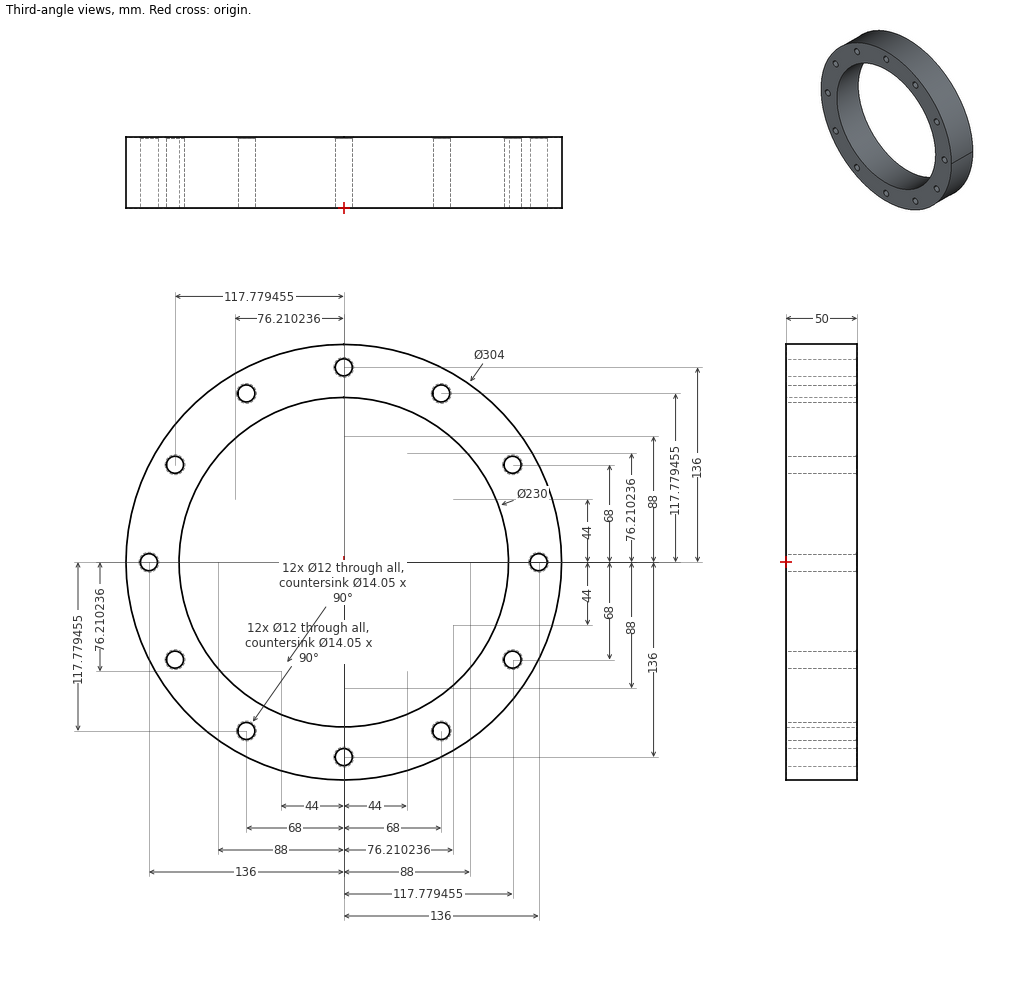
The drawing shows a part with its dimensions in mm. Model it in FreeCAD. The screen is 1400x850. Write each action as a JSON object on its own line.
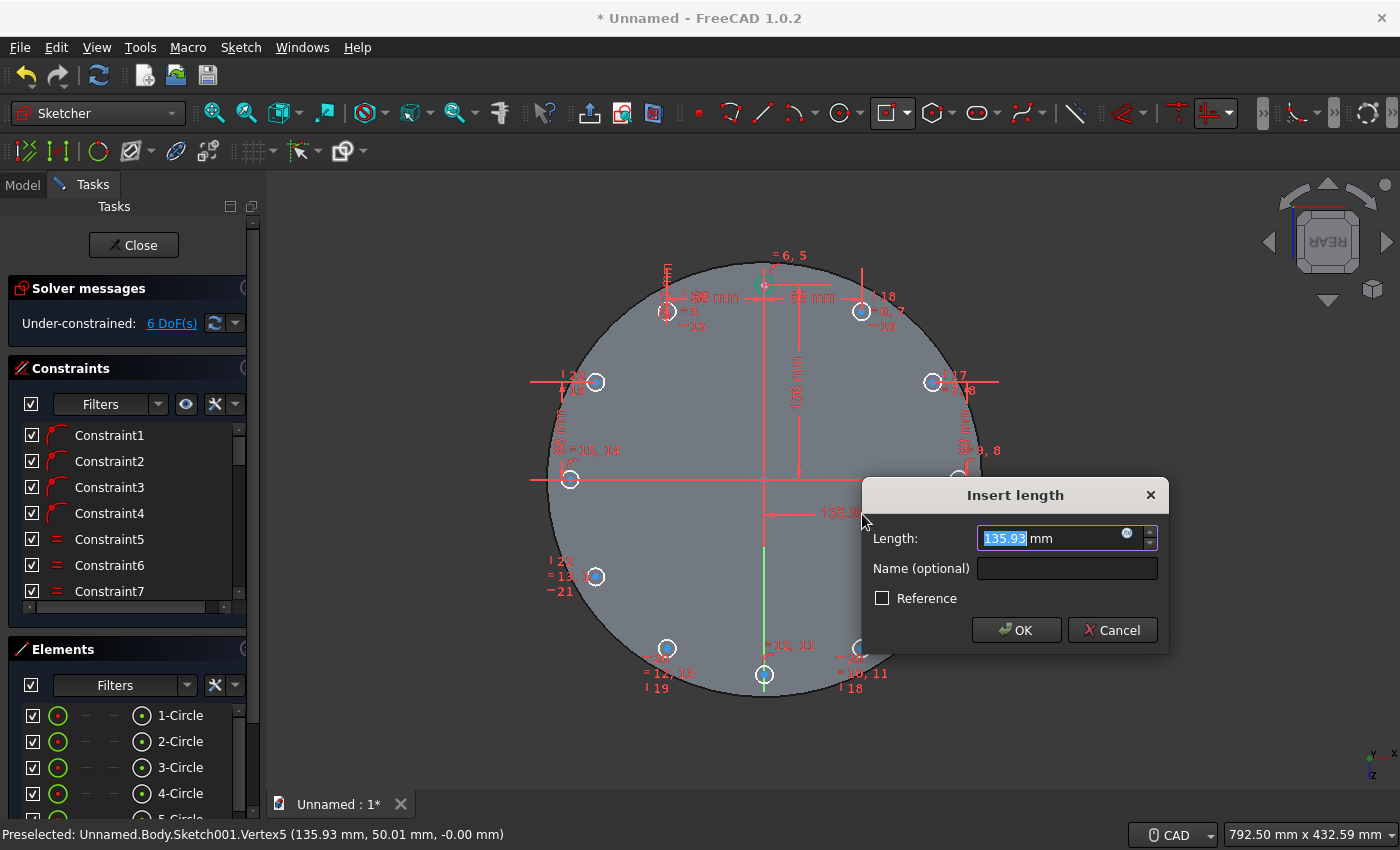
{"action": "type", "text": "136"}
{"action": "key", "text": "Return"}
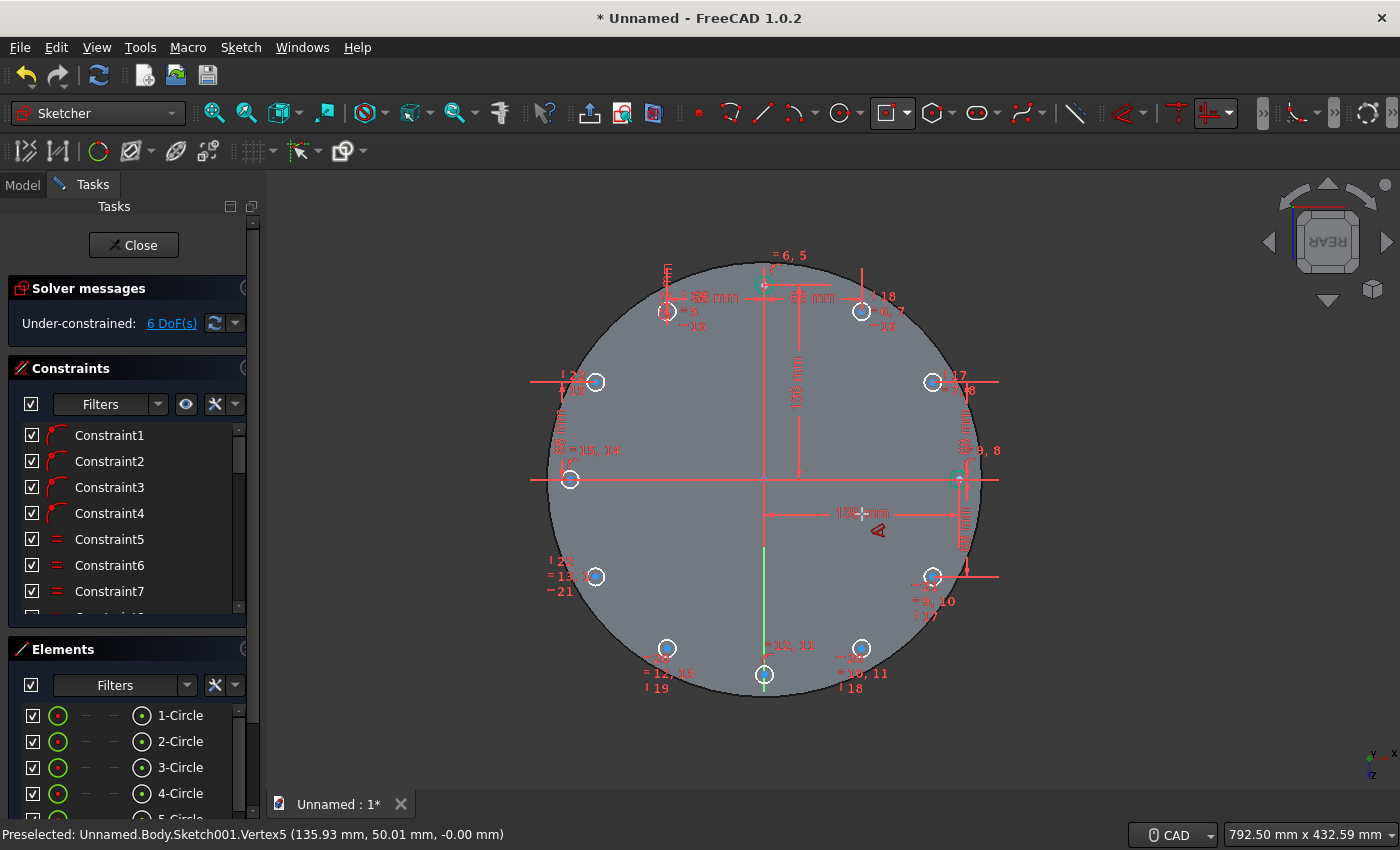
{"action": "left_click", "coordinate": [765, 675]}
{"action": "left_click", "coordinate": [799, 577]}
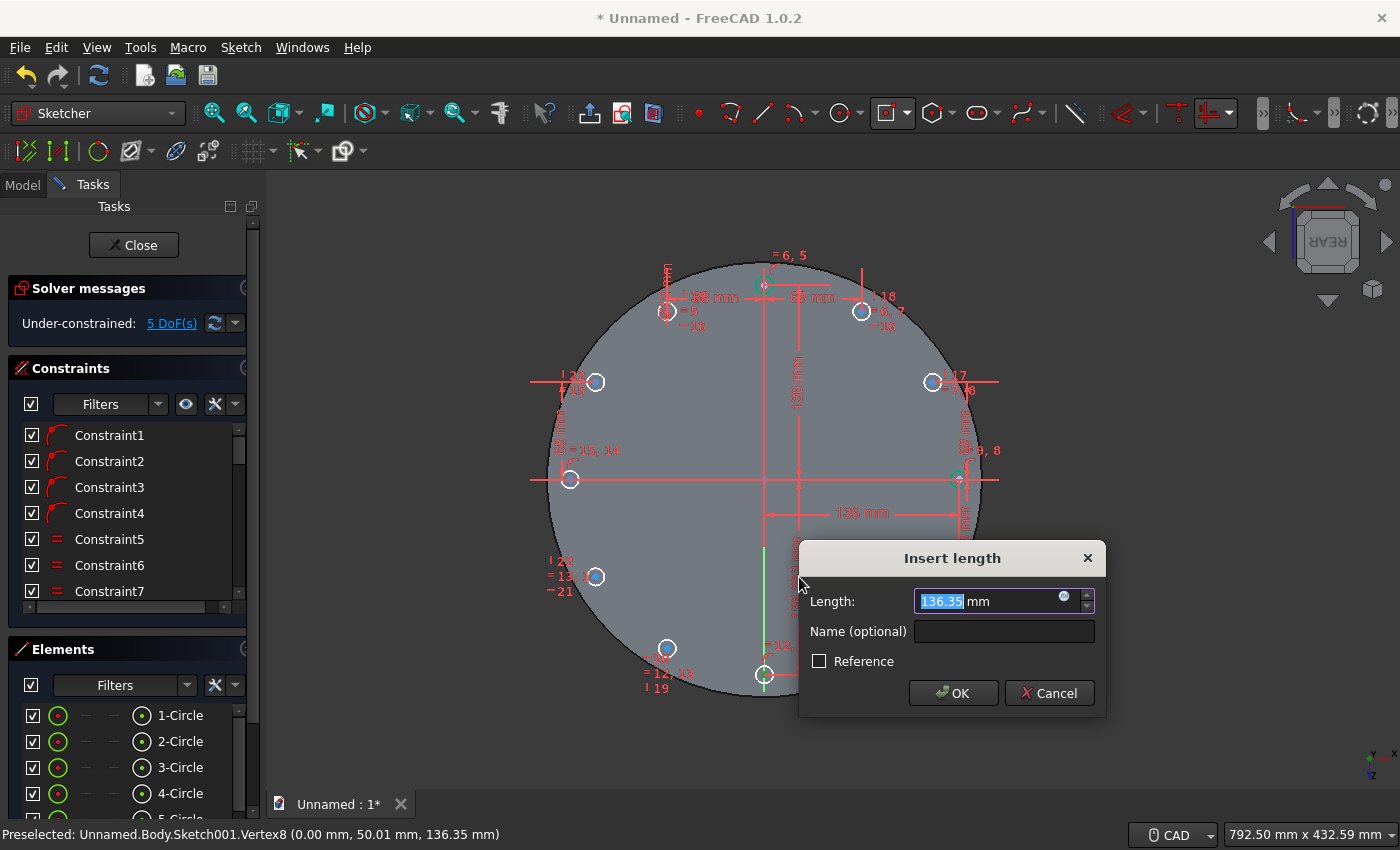
{"action": "type", "text": "136"}
{"action": "key", "text": "Return"}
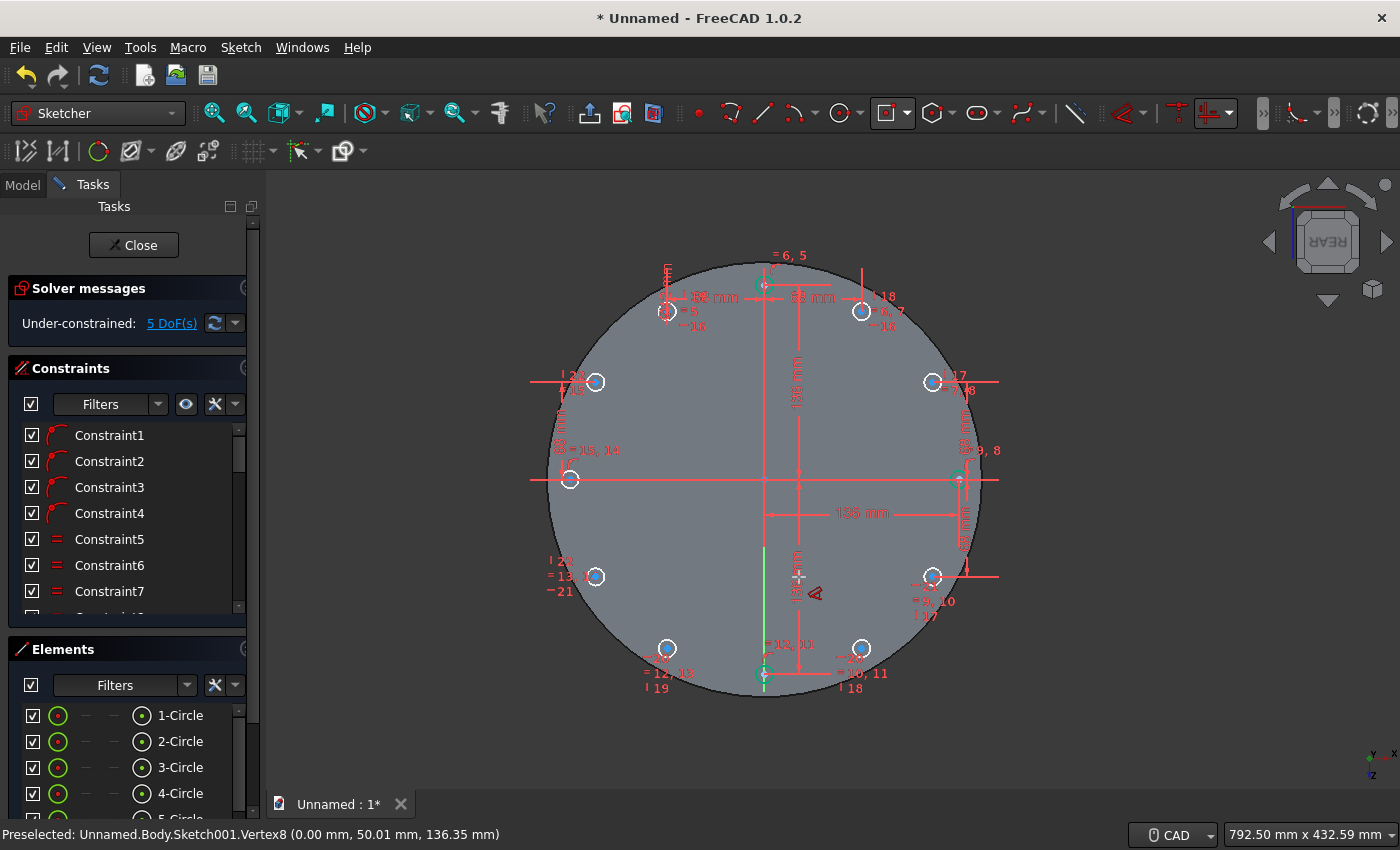
{"action": "left_click", "coordinate": [570, 480]}
{"action": "left_click", "coordinate": [667, 514]}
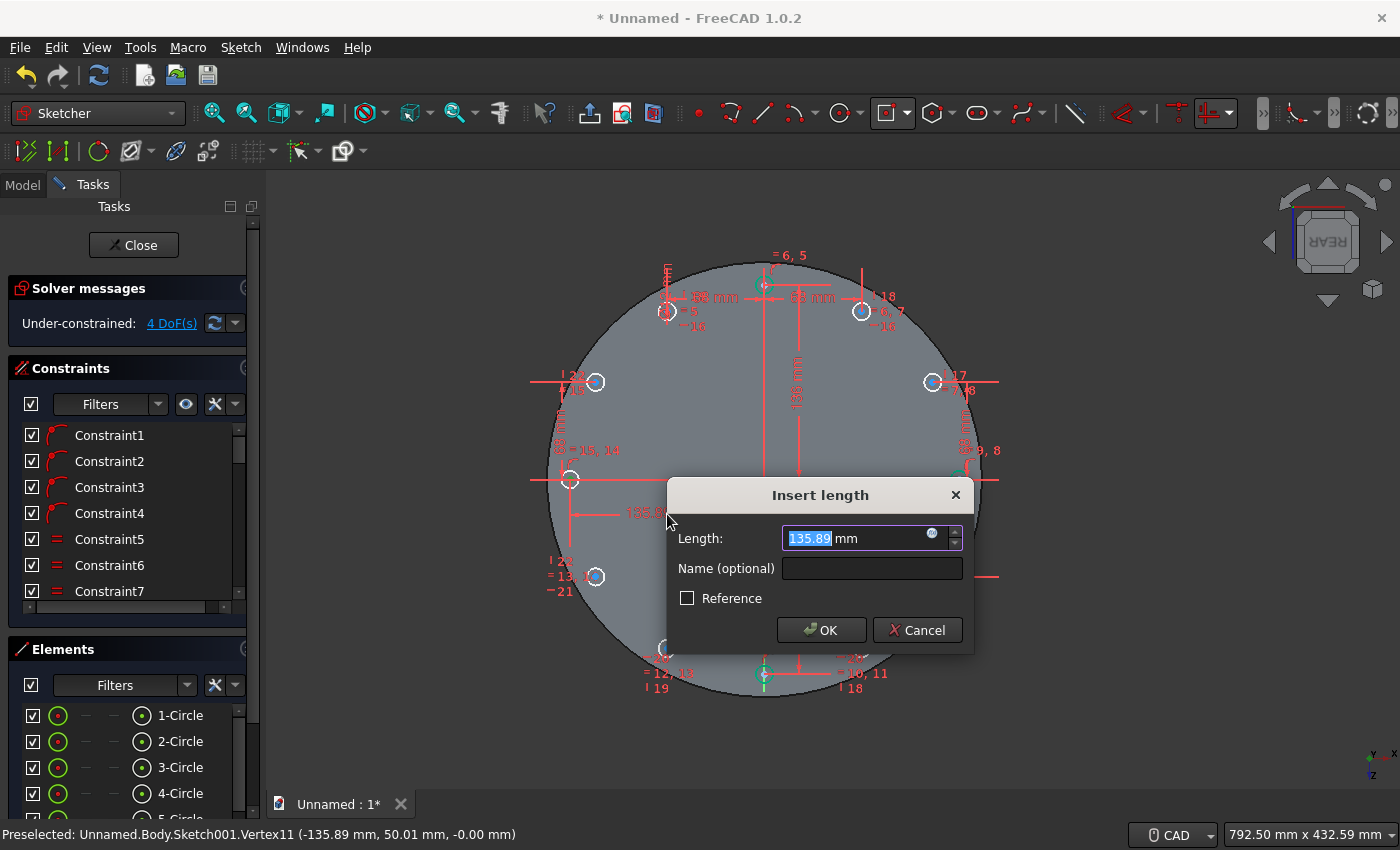
{"action": "type", "text": "136"}
{"action": "key", "text": "Return"}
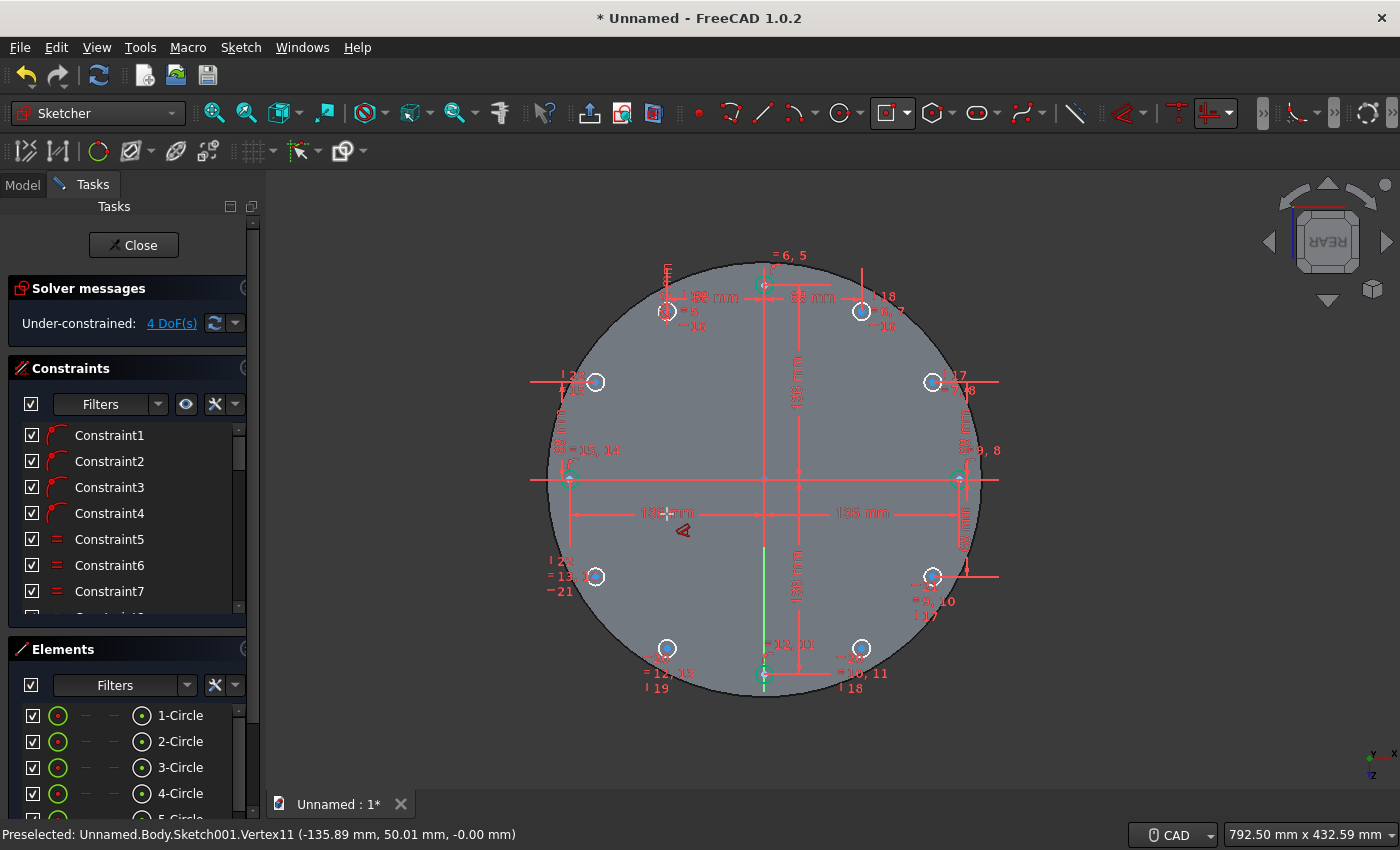
{"action": "left_click", "coordinate": [667, 312]}
{"action": "left_click", "coordinate": [633, 396]}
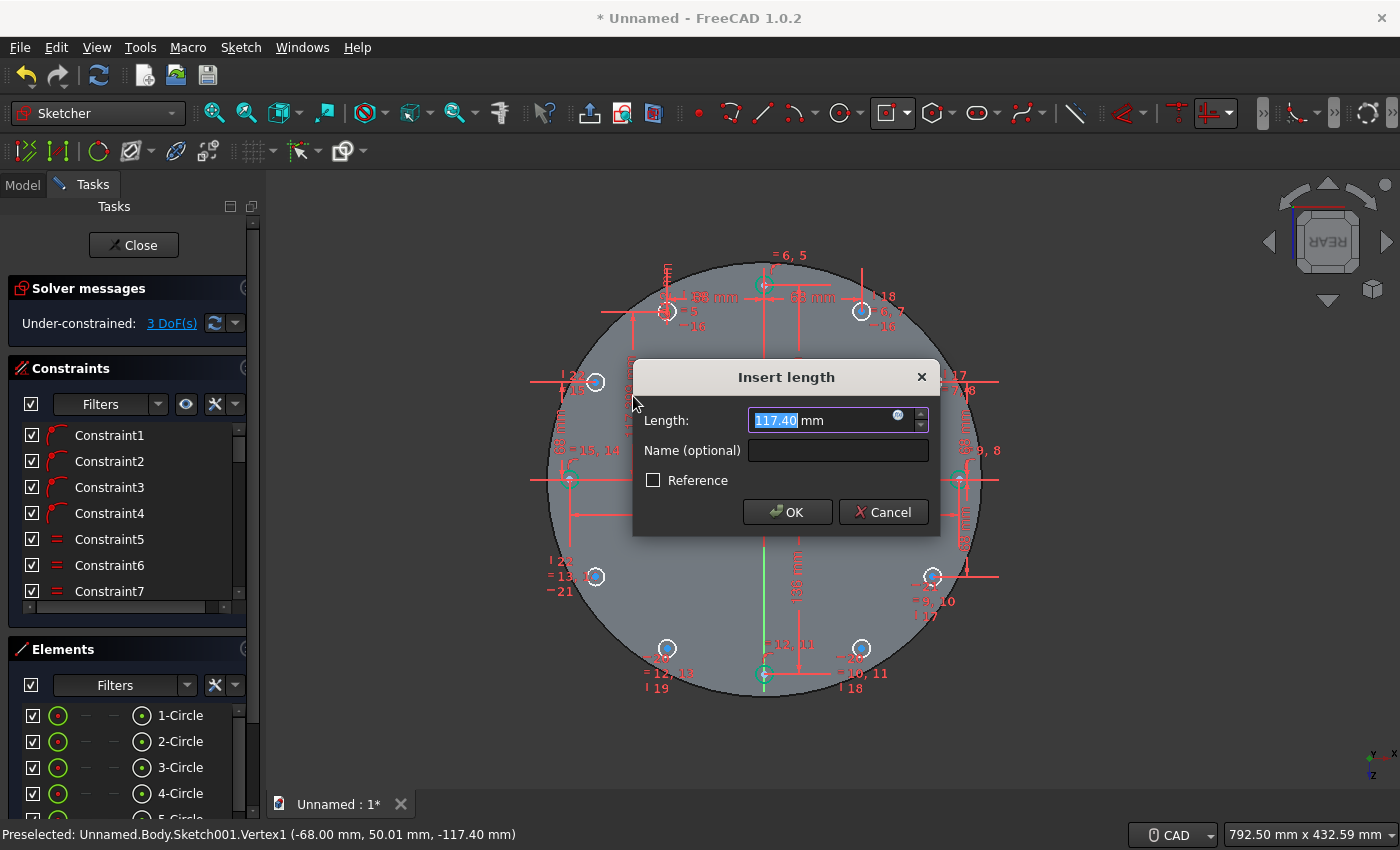
{"action": "type", "text": "117.779455"}
{"action": "key", "text": "Return"}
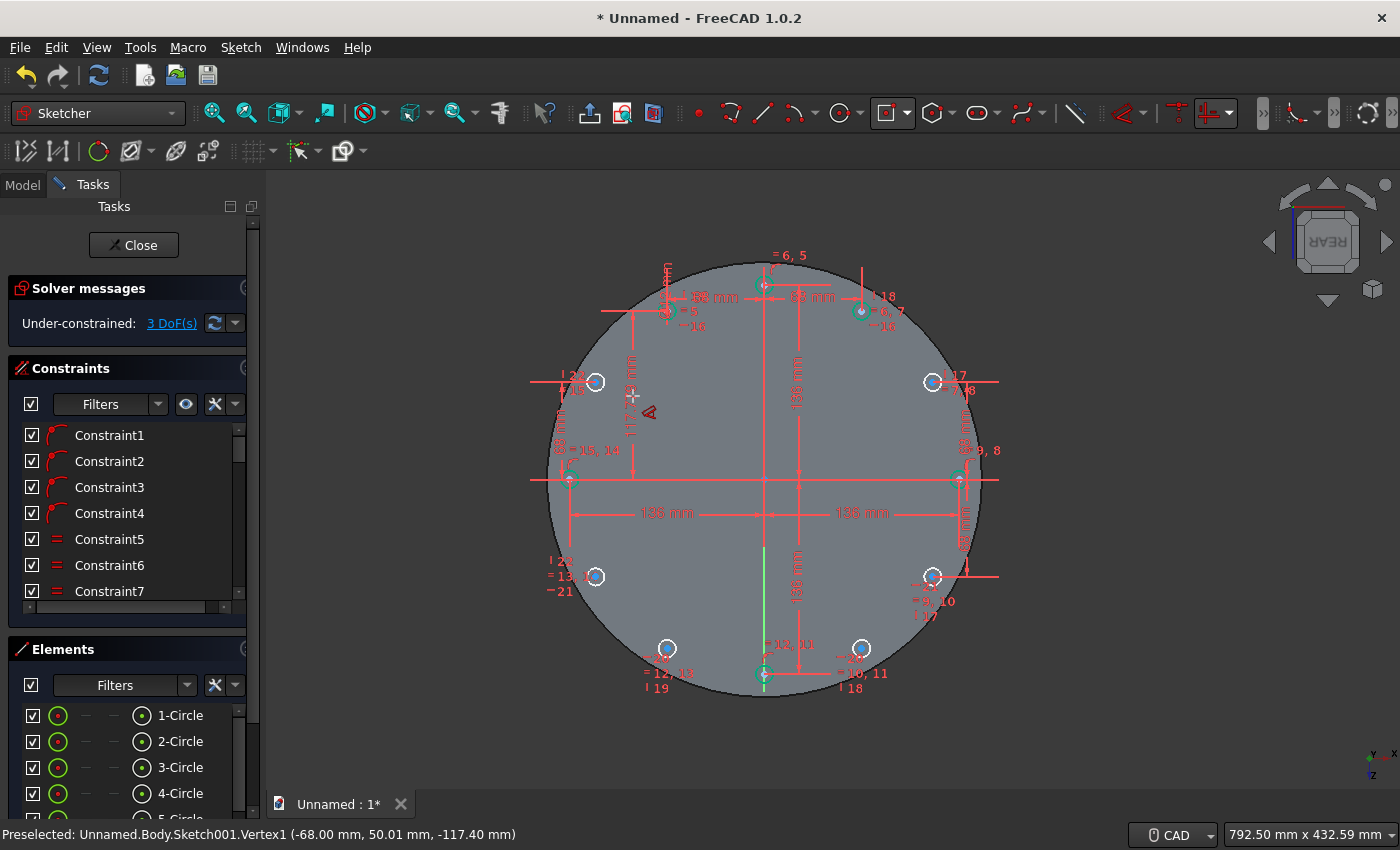
{"action": "left_click", "coordinate": [933, 382]}
{"action": "left_click", "coordinate": [849, 348]}